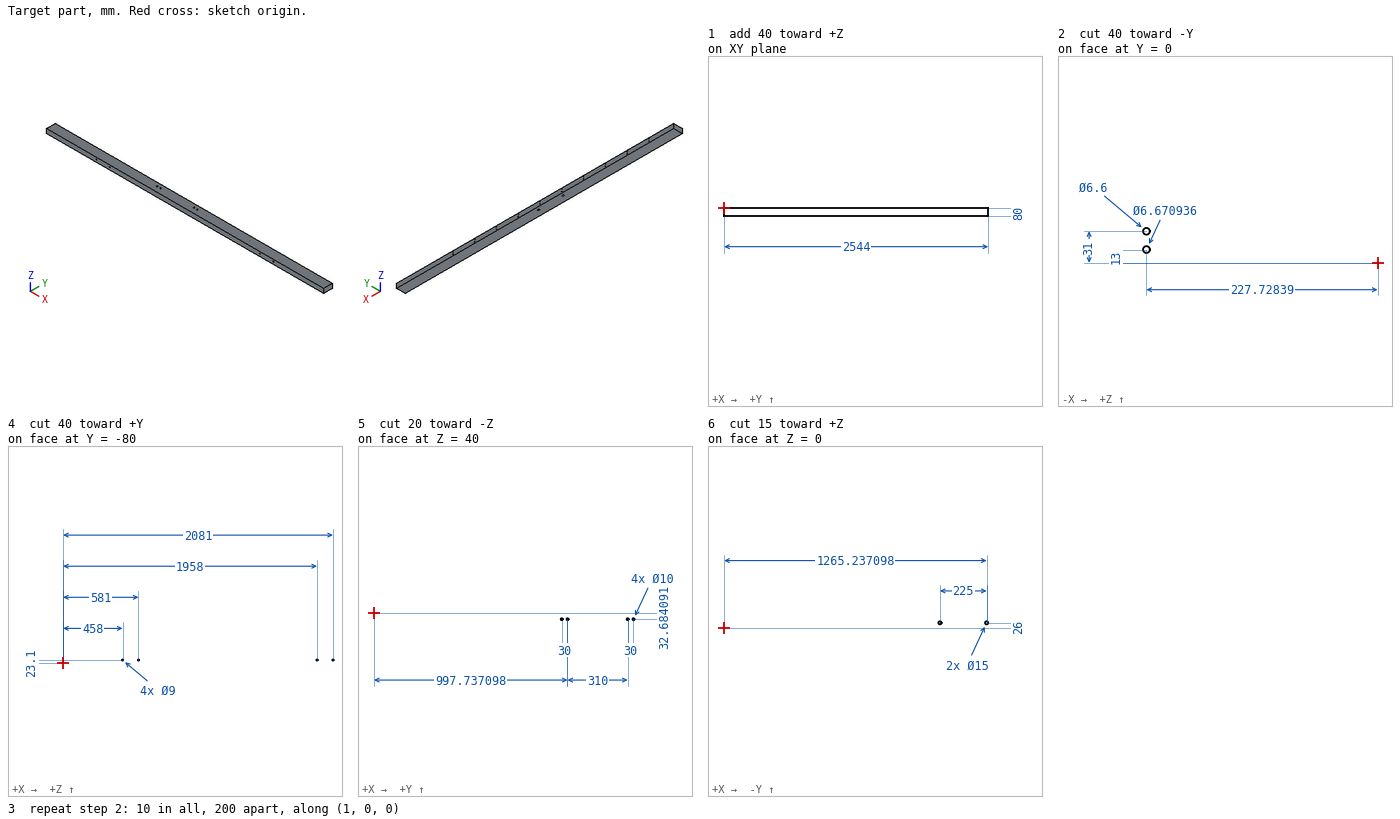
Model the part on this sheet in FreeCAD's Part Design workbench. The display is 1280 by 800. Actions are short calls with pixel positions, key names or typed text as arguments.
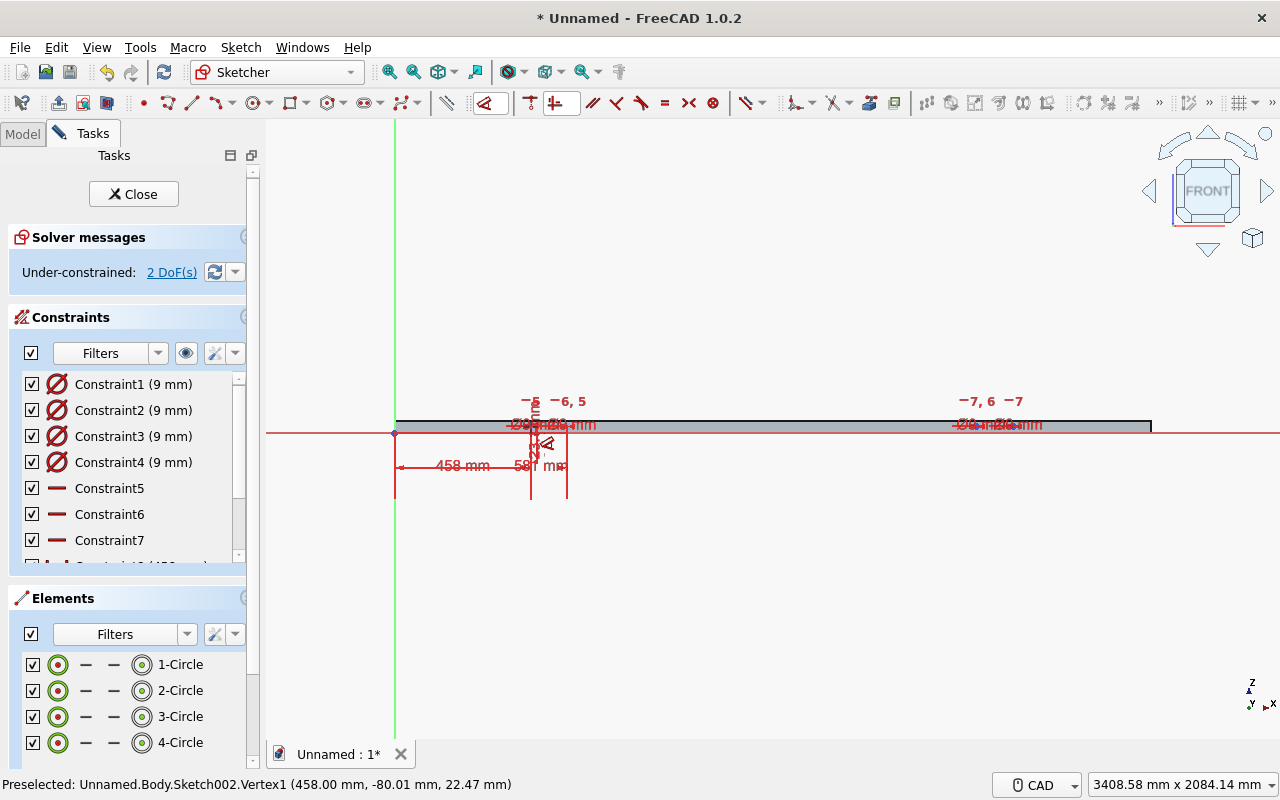
click(977, 426)
click(686, 467)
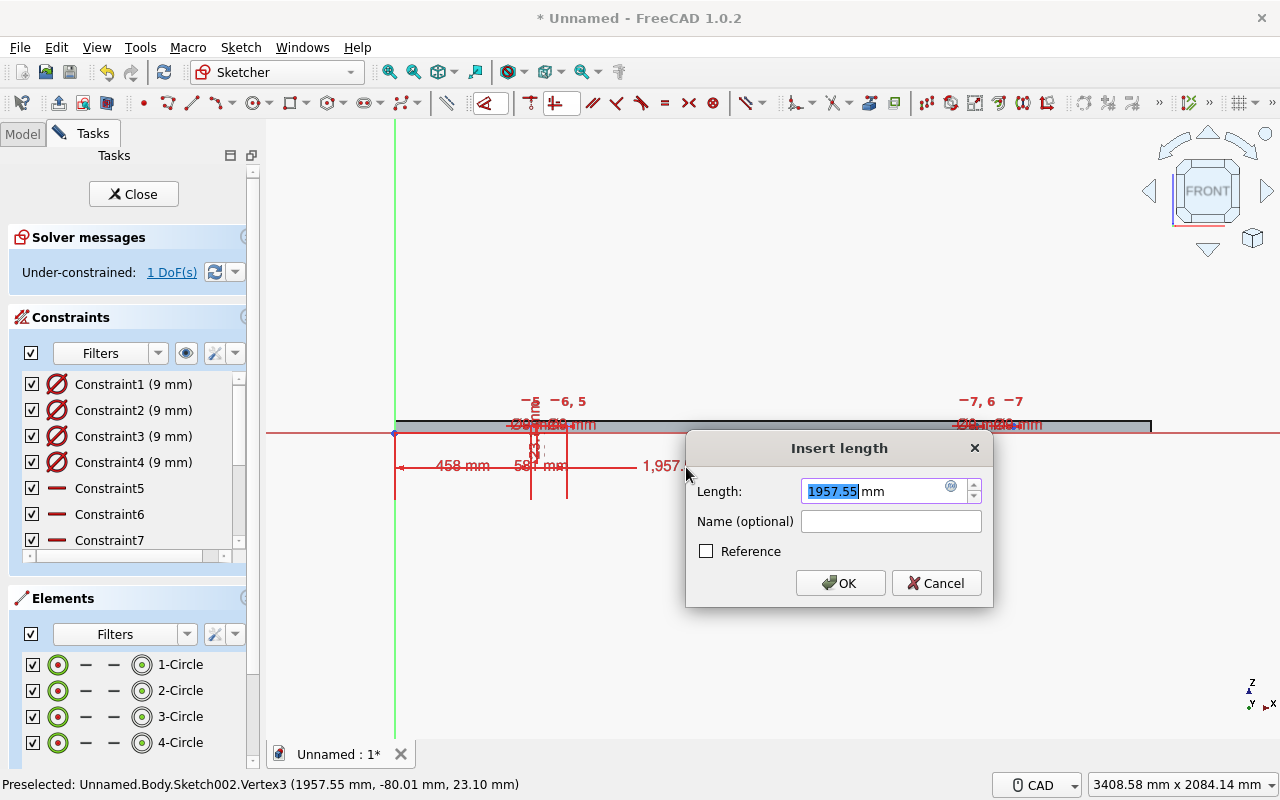
text(1958)
key(Return)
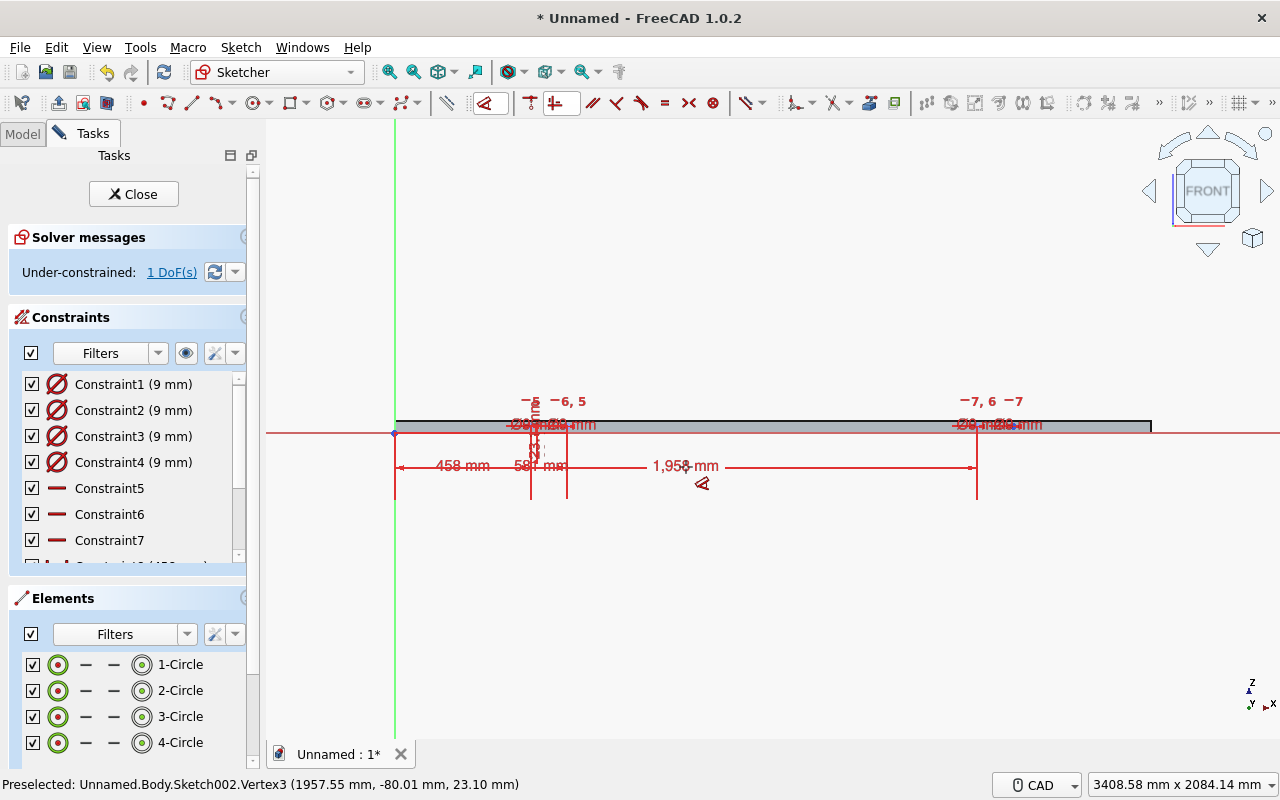
click(1014, 426)
click(847, 467)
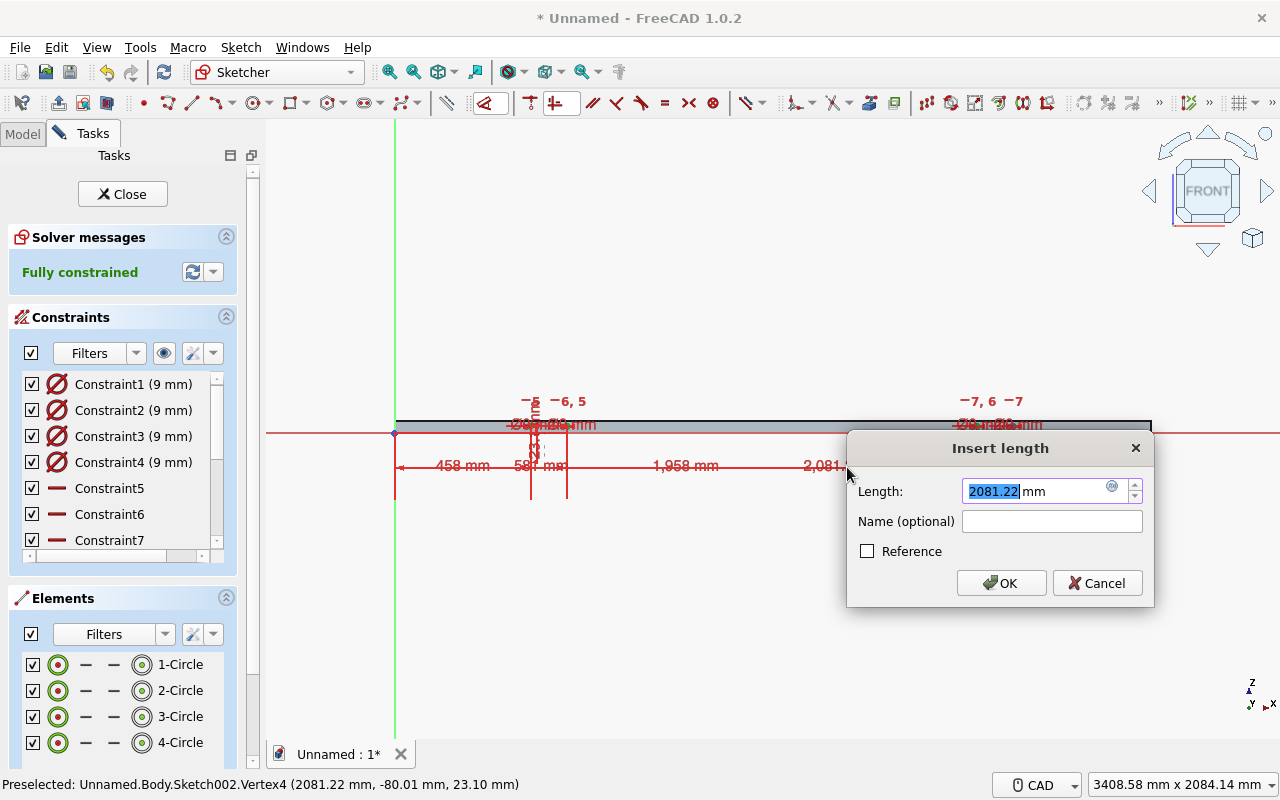
text(2081)
key(Return)
key(Escape)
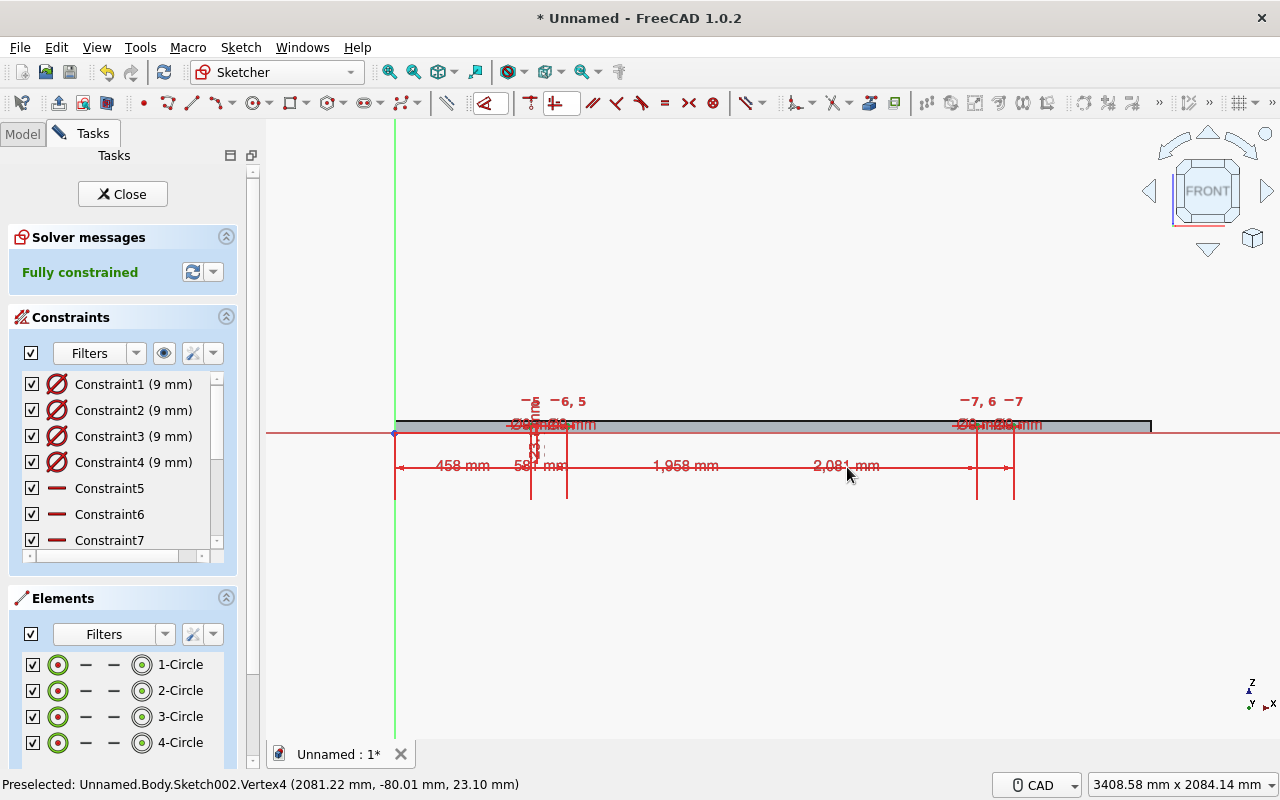
click(123, 194)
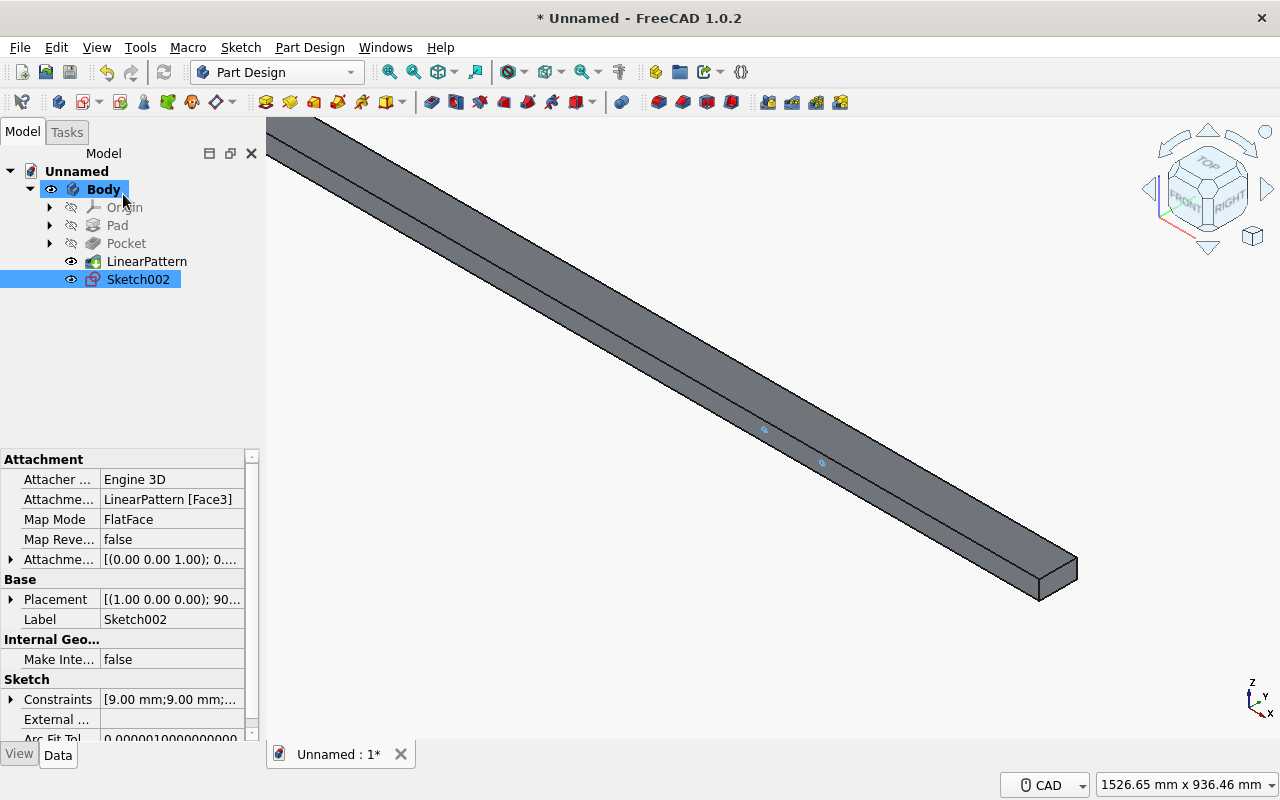
click(432, 102)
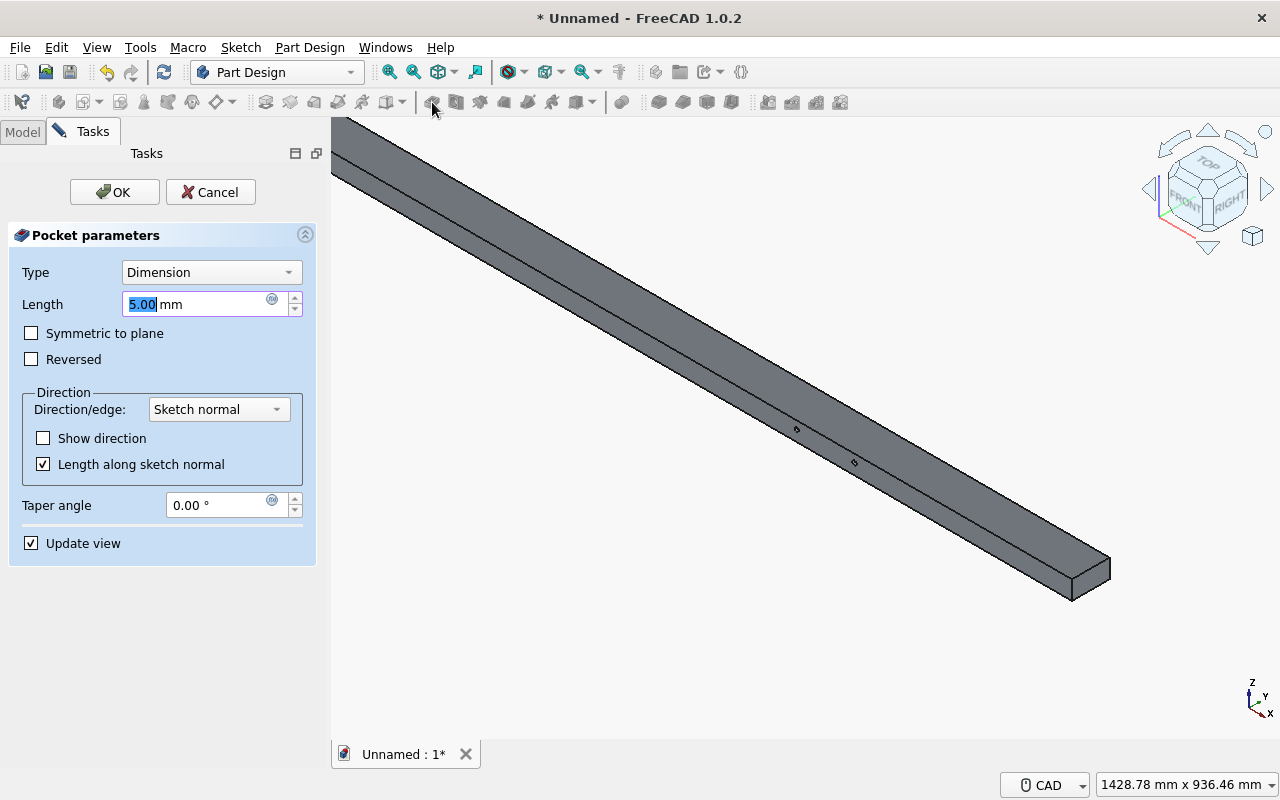
text(40)
key(Tab)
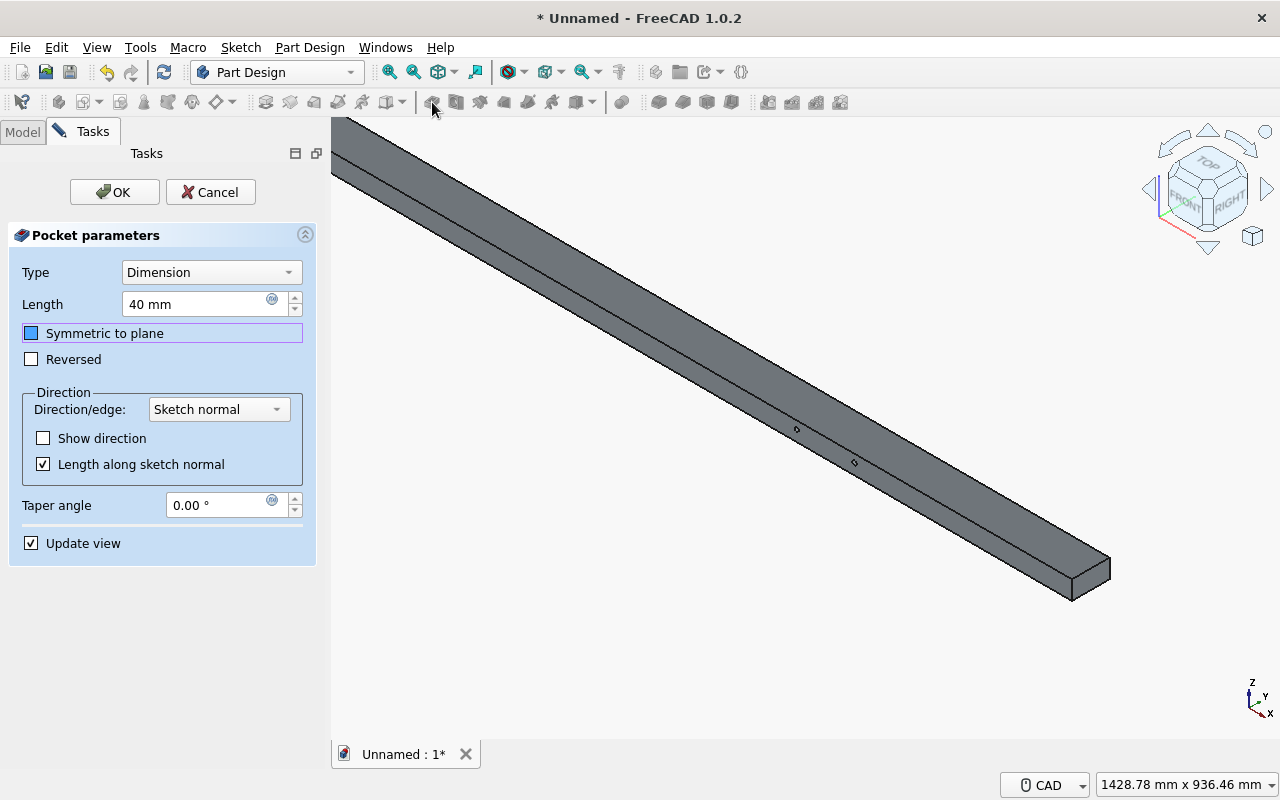
click(115, 192)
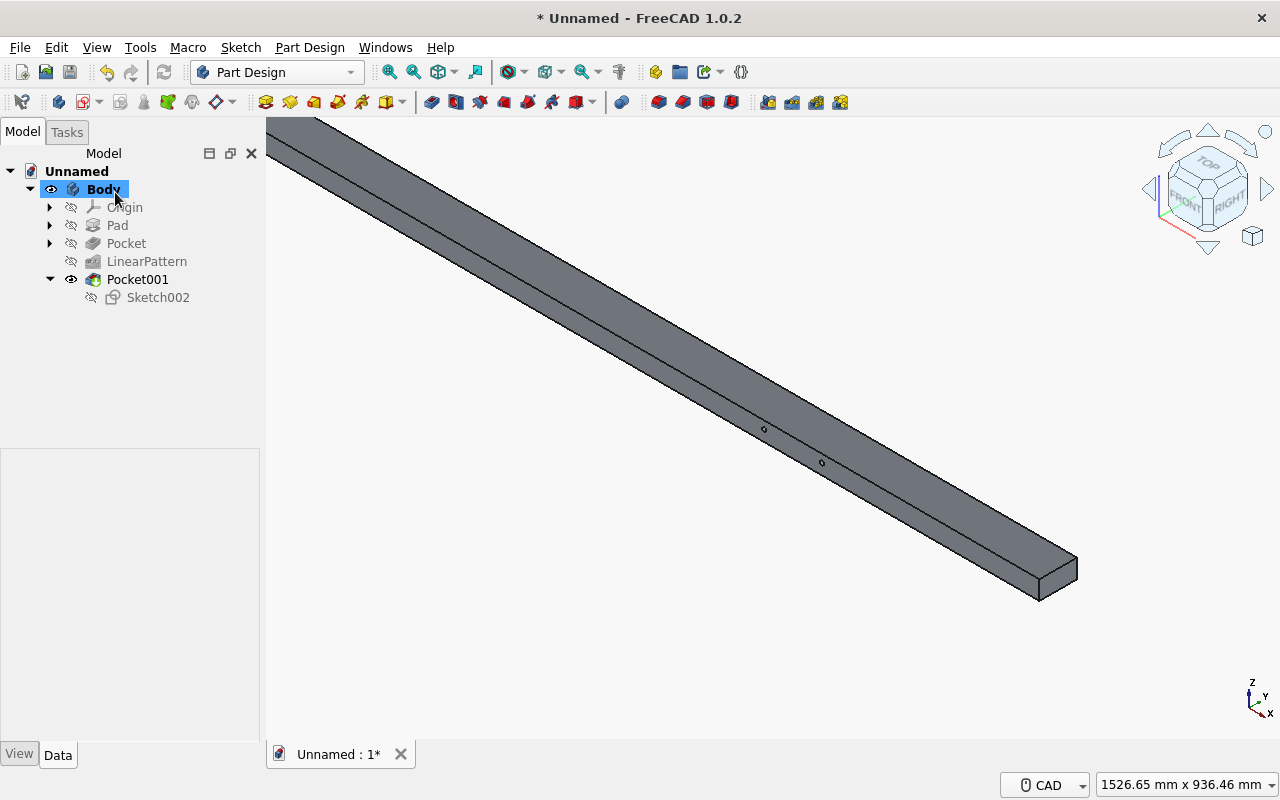
key(v)
key(f)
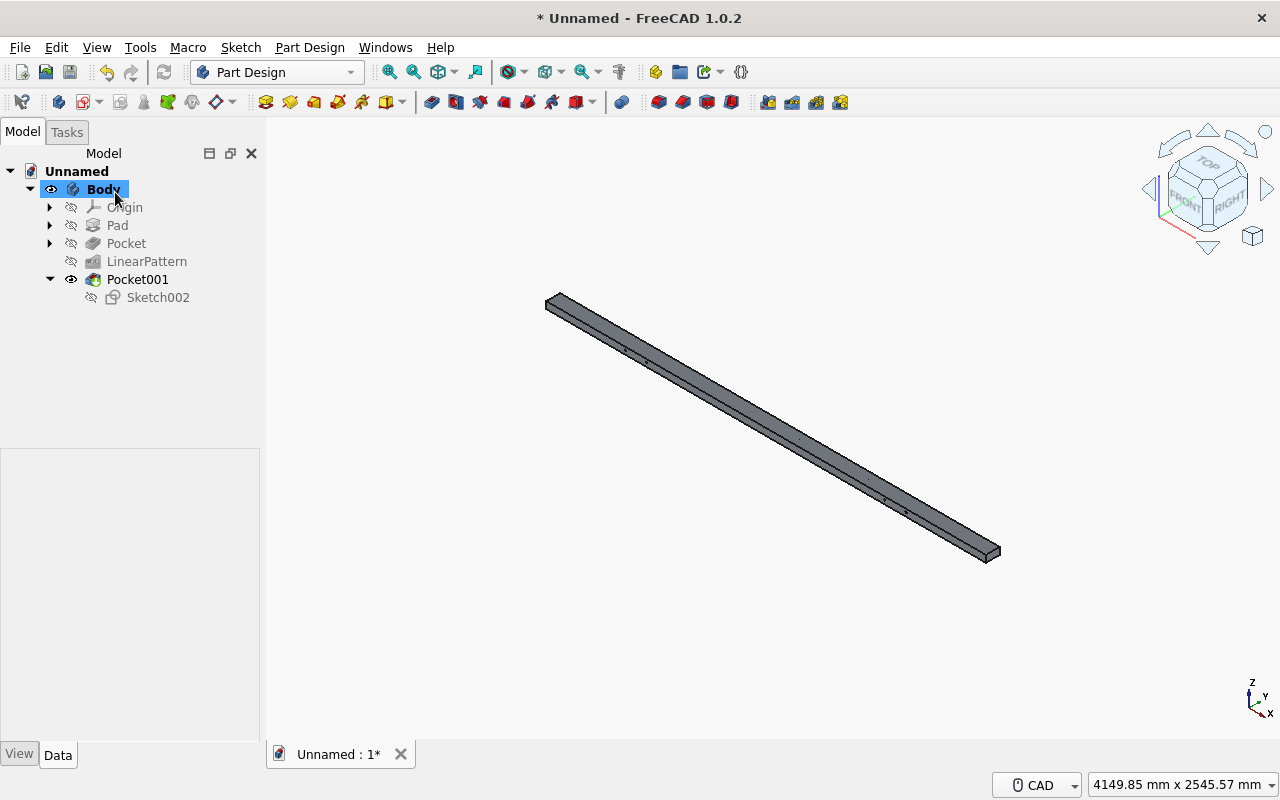
key(2)